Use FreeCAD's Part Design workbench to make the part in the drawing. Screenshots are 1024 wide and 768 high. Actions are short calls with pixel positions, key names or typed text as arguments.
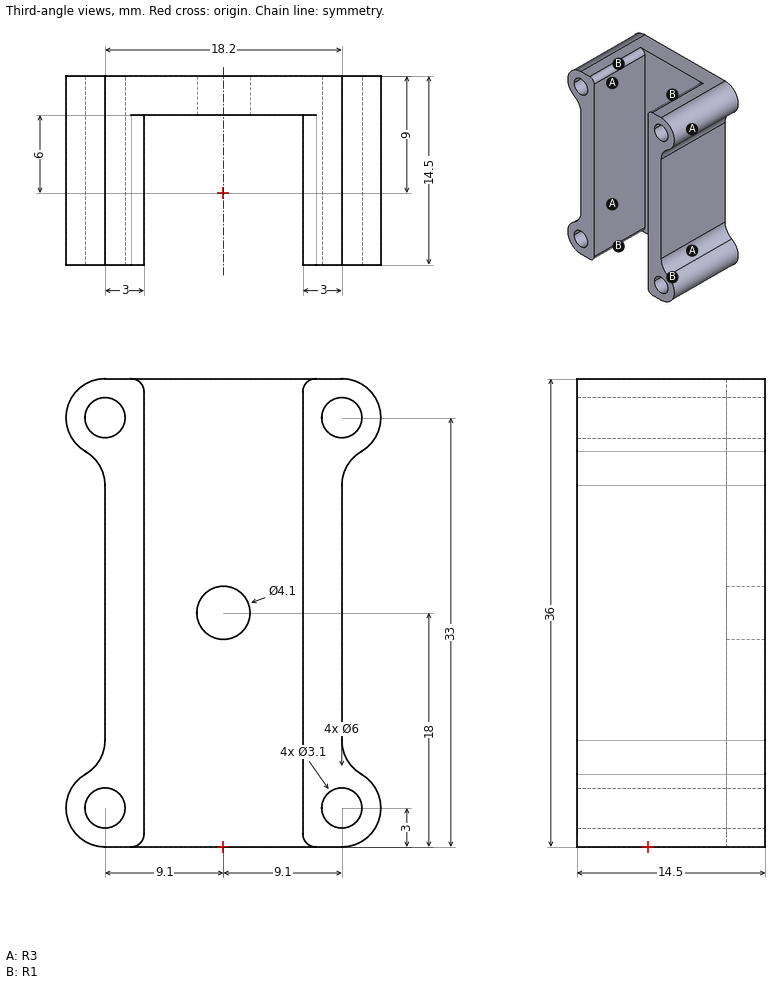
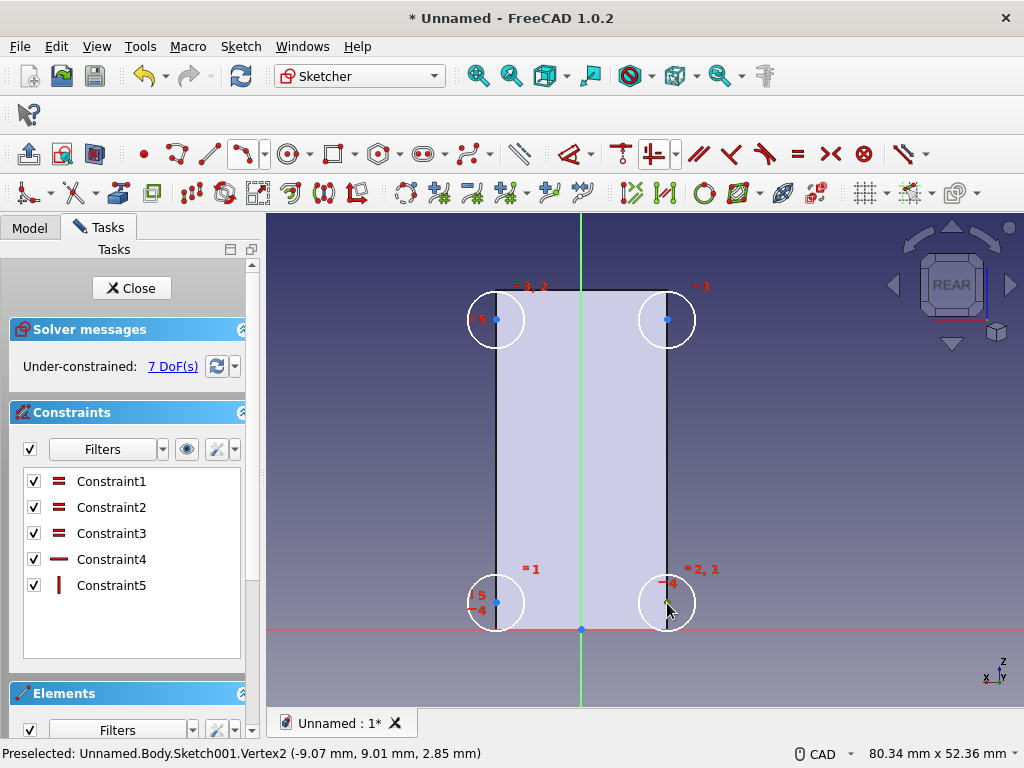
click(667, 320)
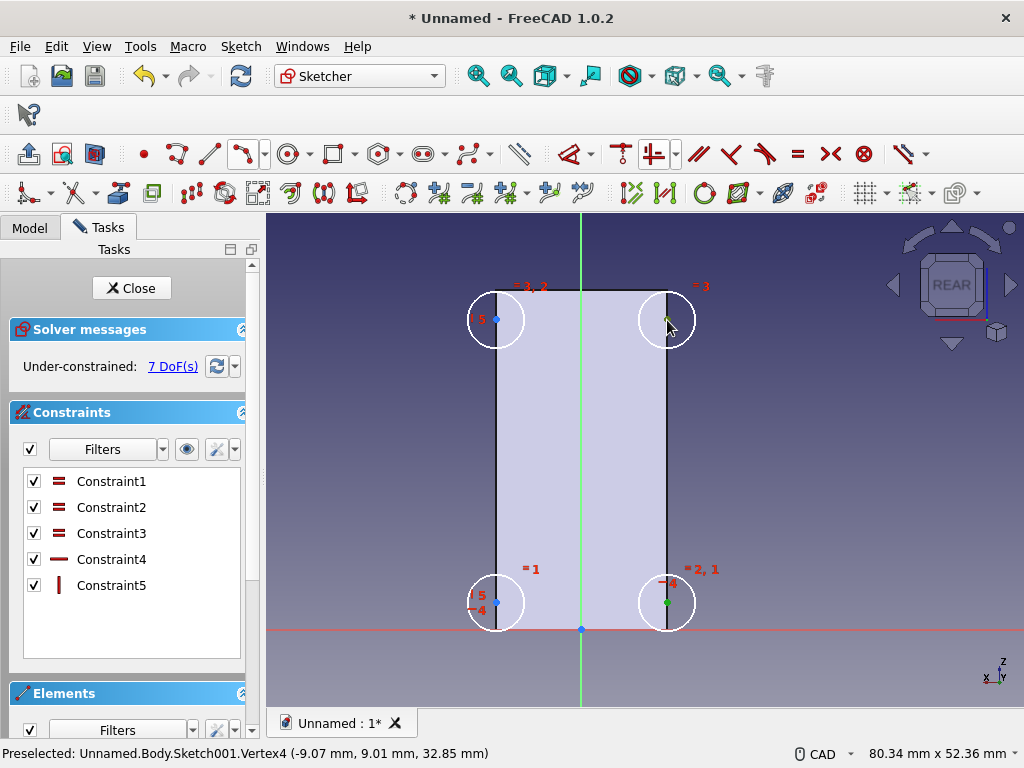
key(v)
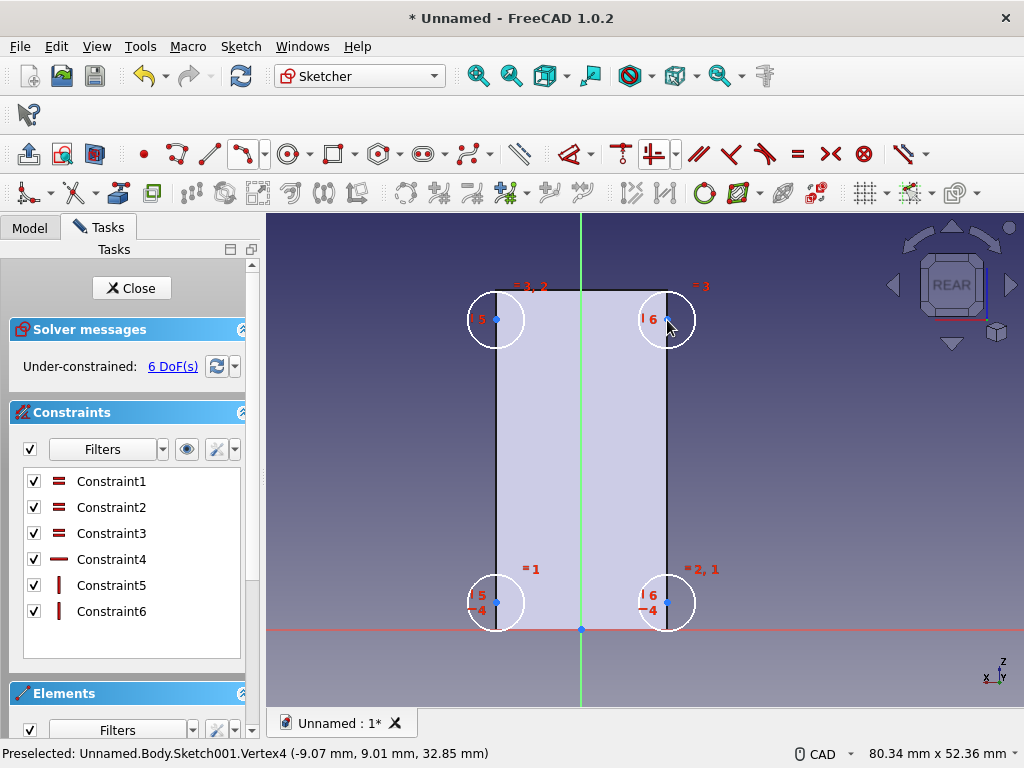
click(496, 320)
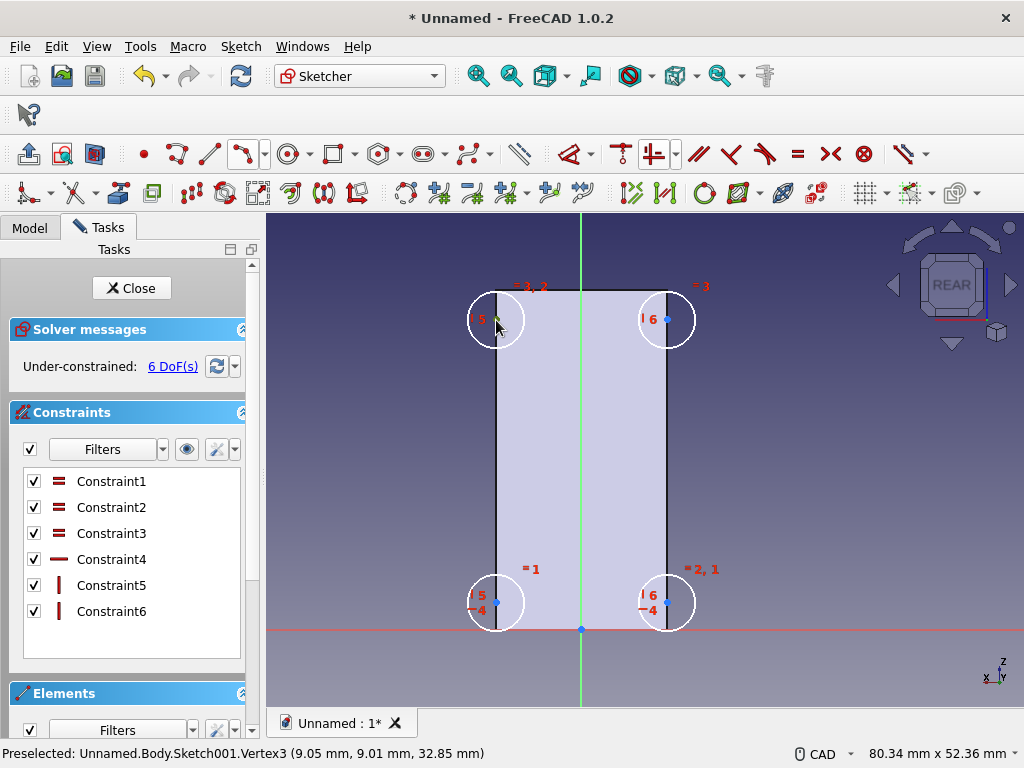
click(667, 320)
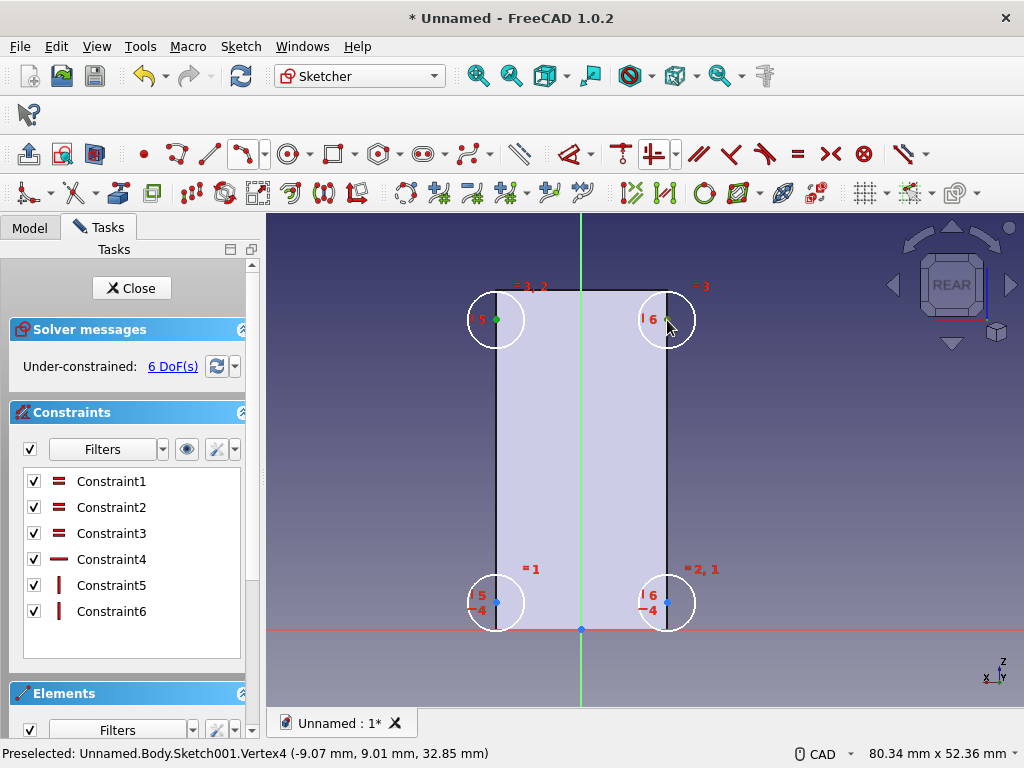
click(676, 154)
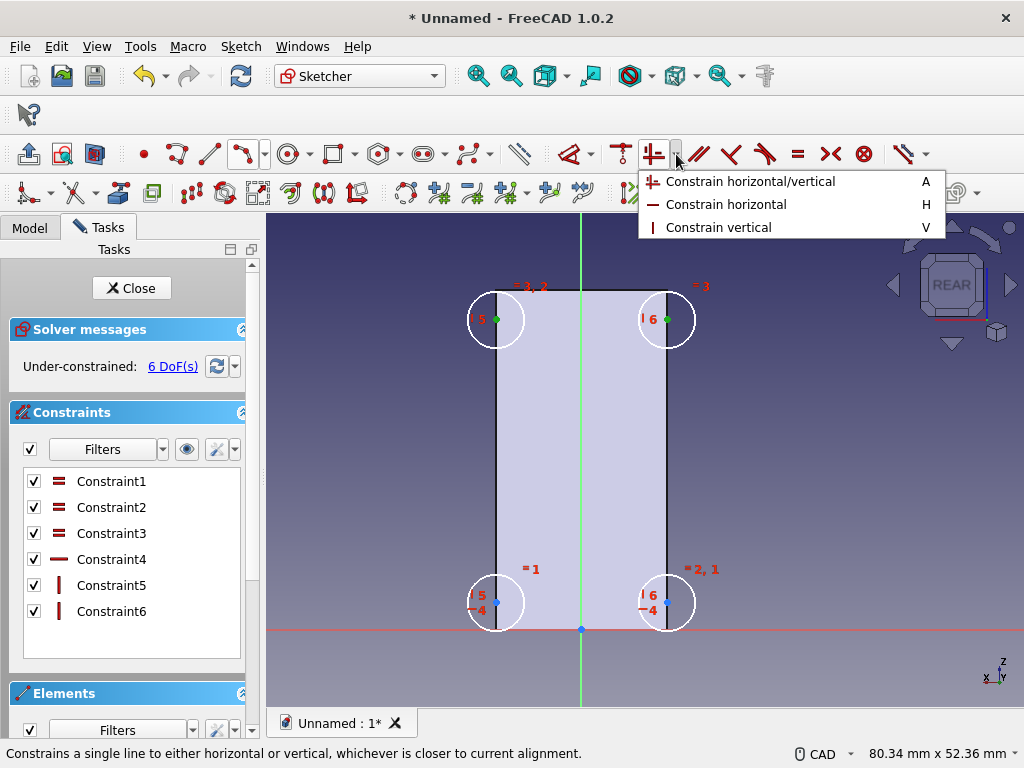
click(792, 204)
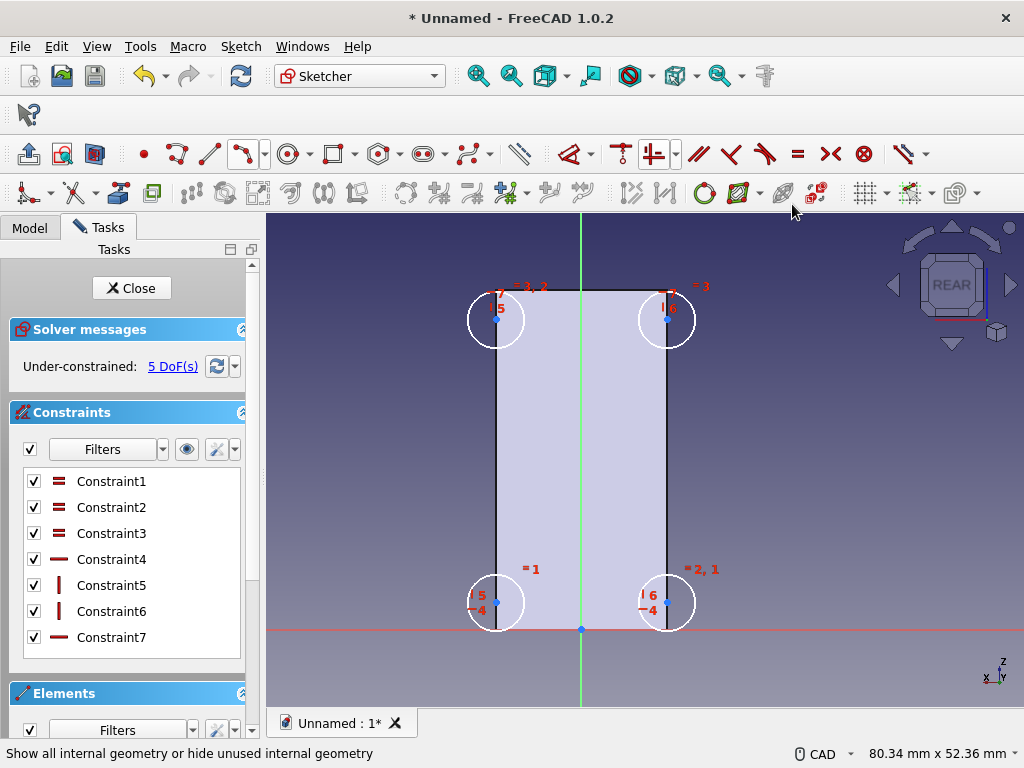
click(568, 154)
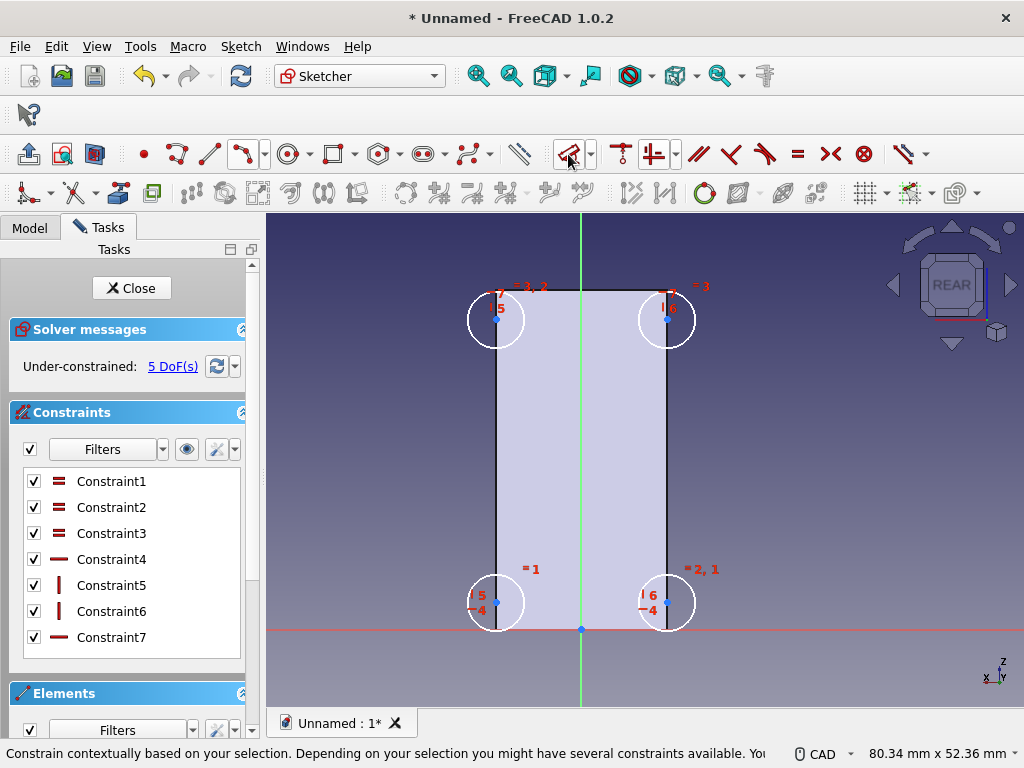
click(516, 583)
click(539, 560)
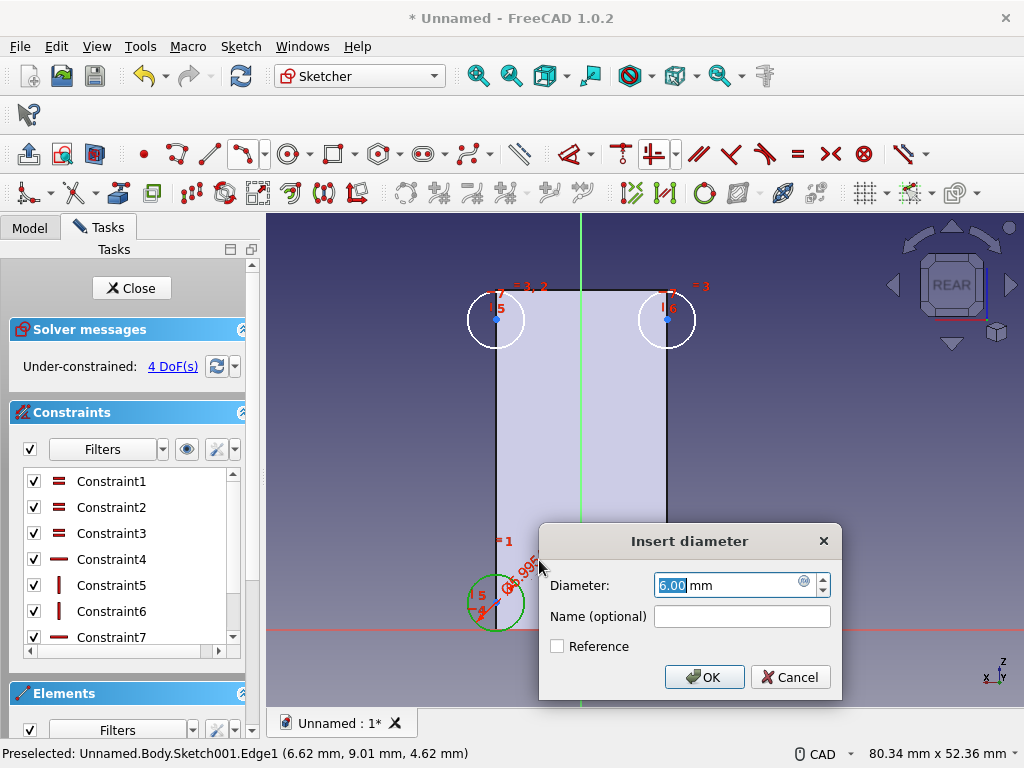
text(6)
key(Return)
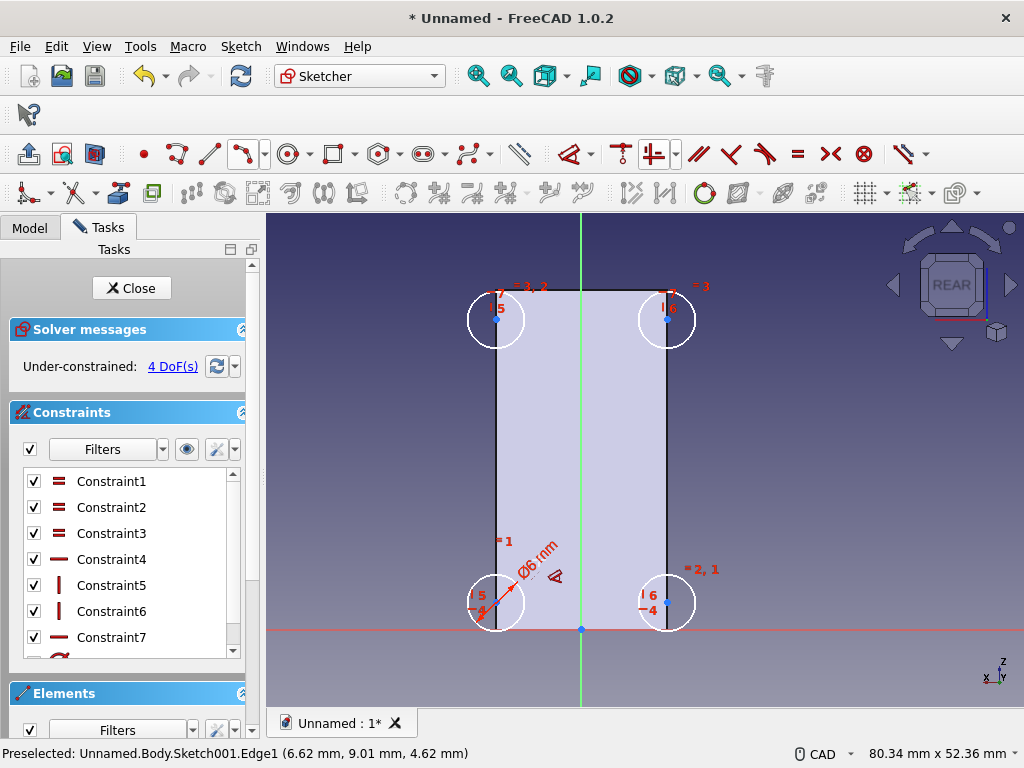
scroll(496, 603, up, 2)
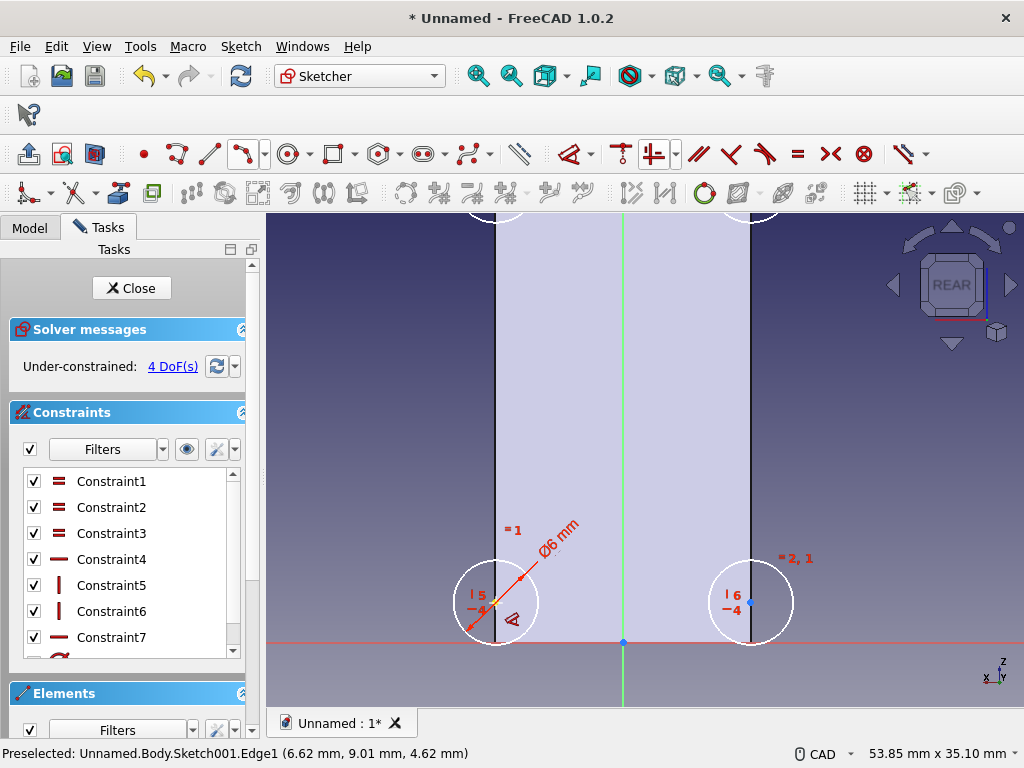
click(496, 603)
click(657, 623)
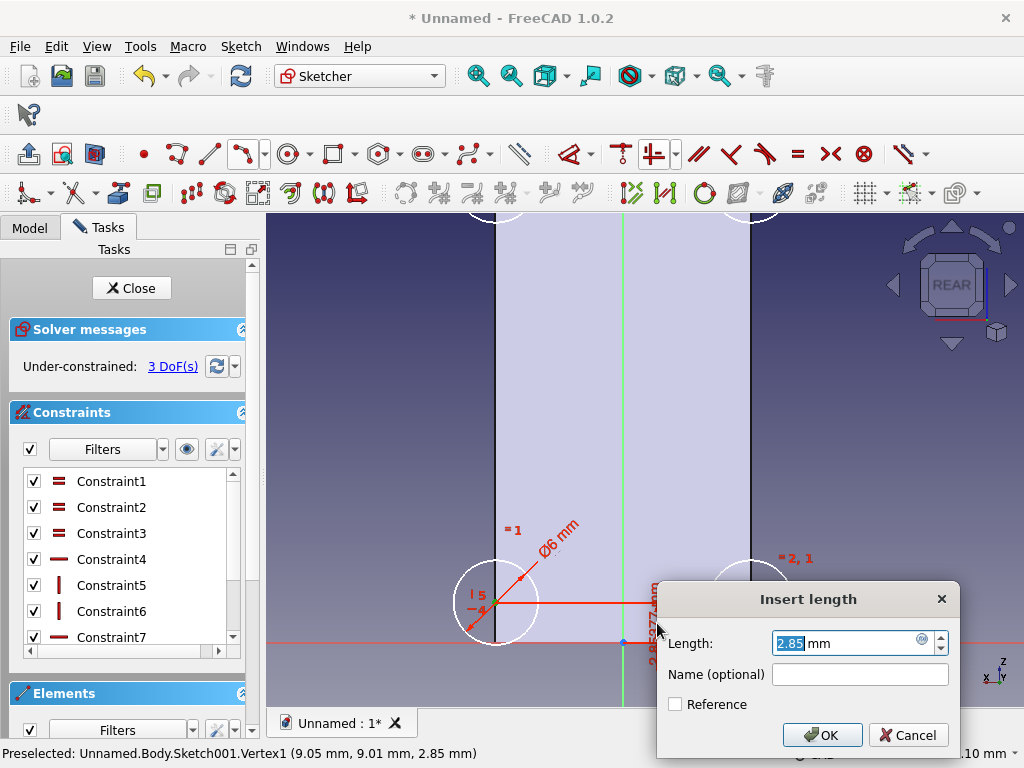
text(3)
key(Return)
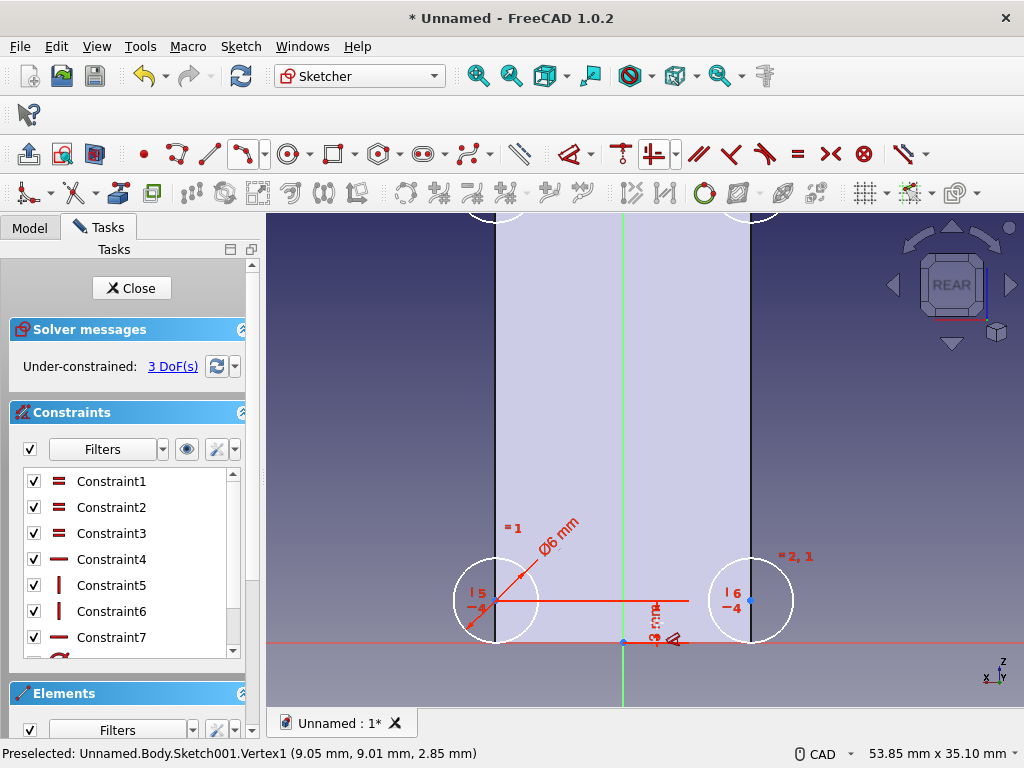
scroll(481, 604, down, 2)